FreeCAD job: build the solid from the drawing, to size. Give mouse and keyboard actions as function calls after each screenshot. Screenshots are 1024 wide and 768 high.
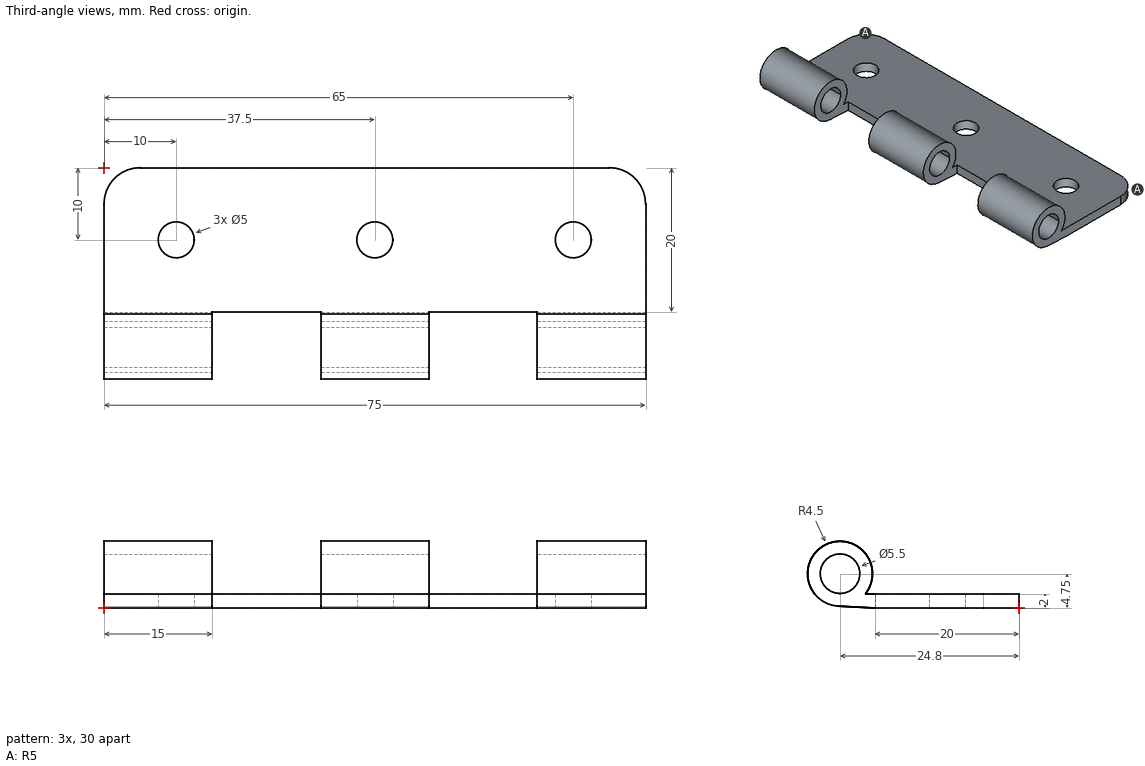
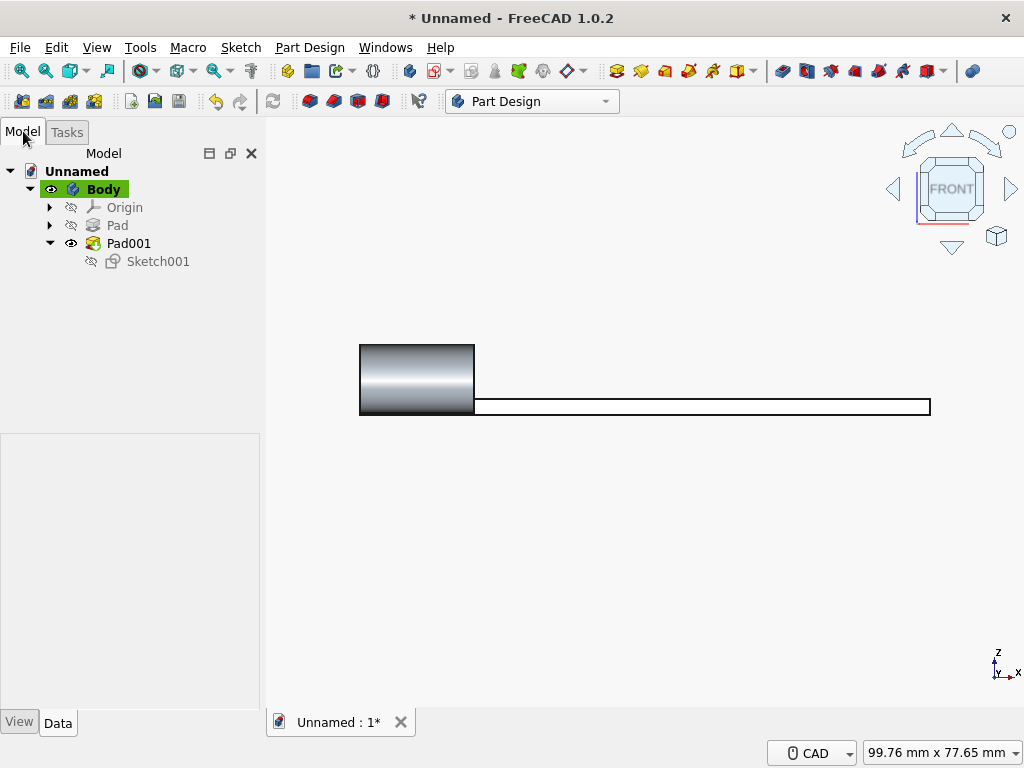
click(116, 243)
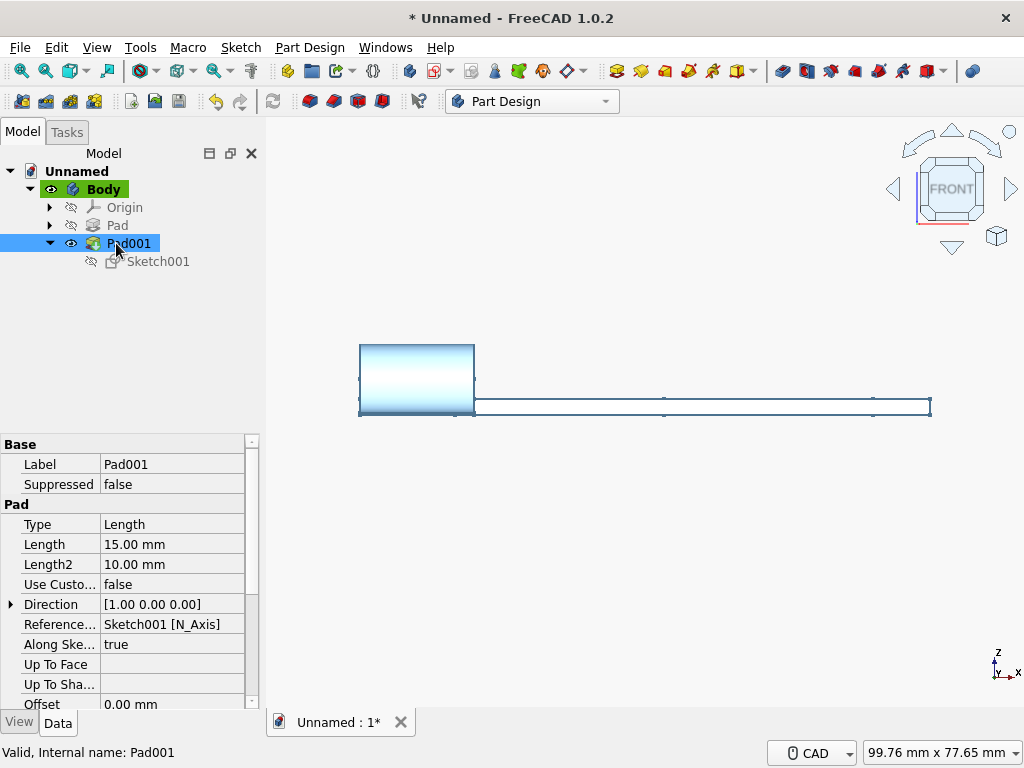
click(46, 102)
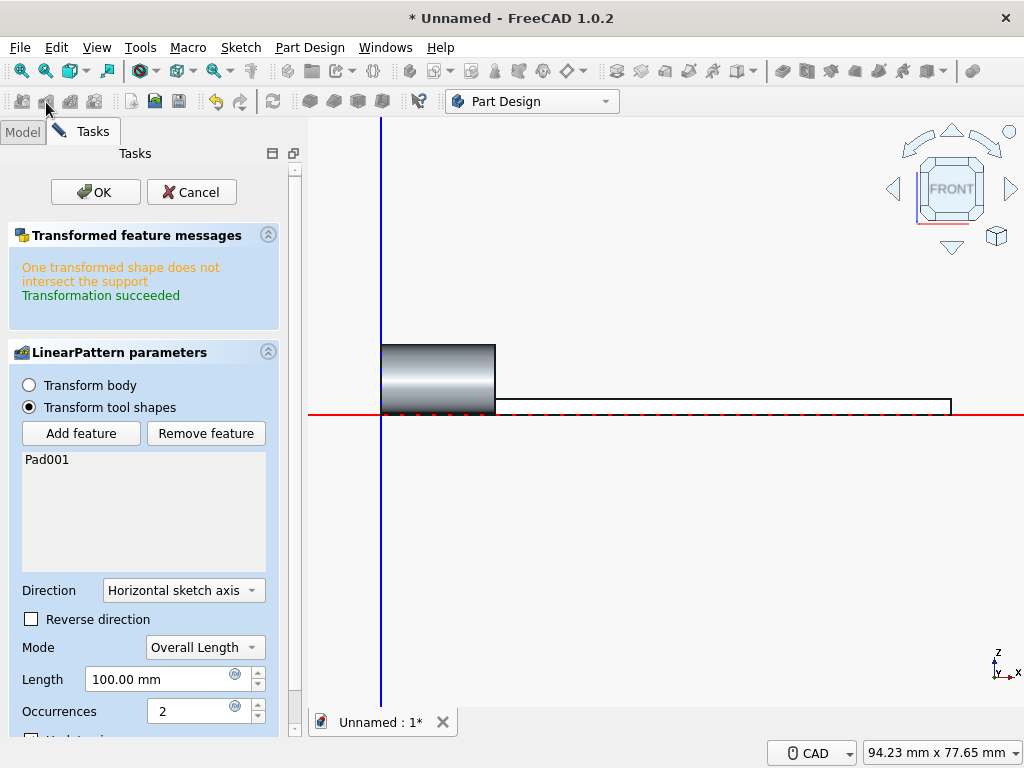
click(184, 590)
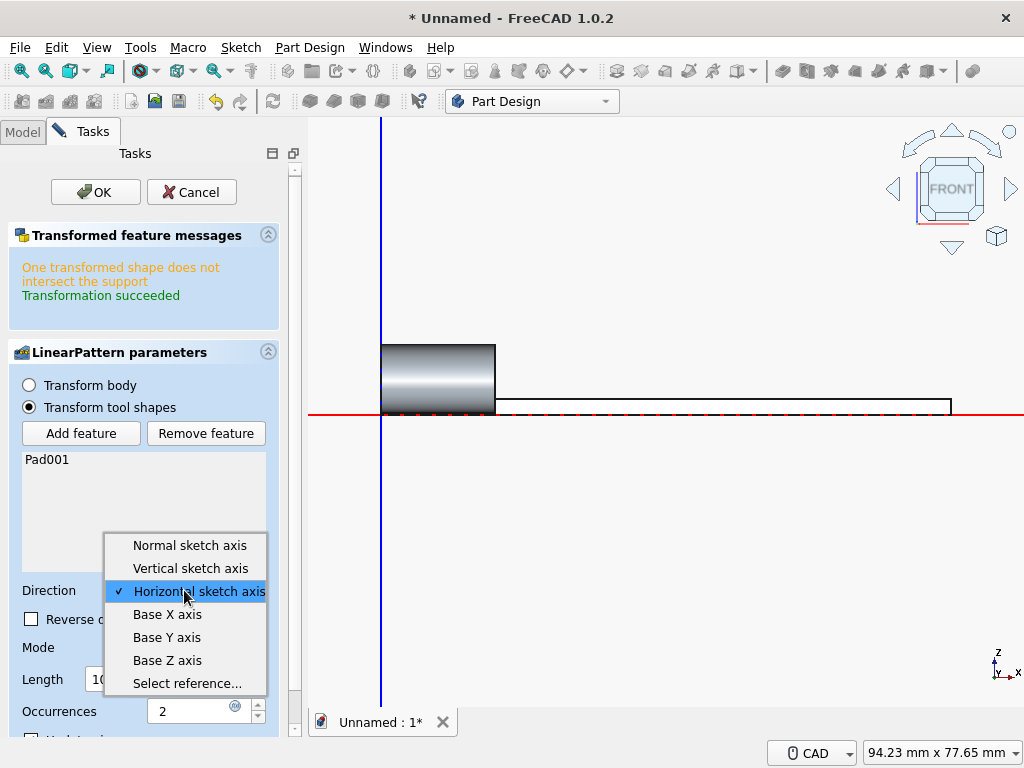
click(184, 614)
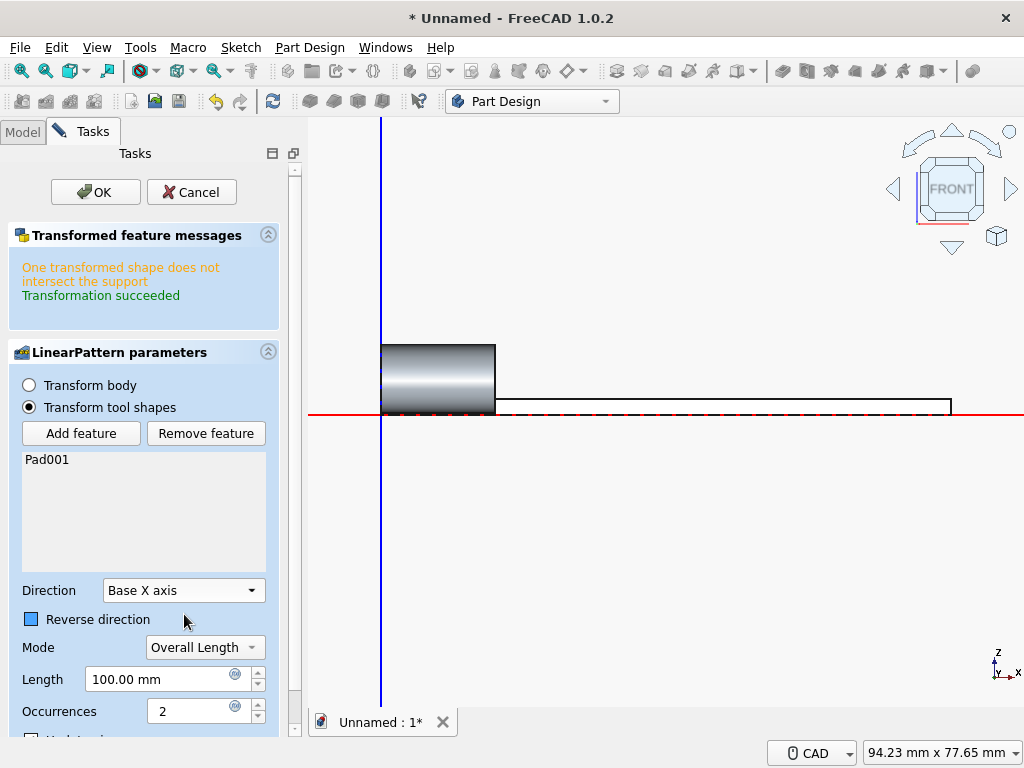
click(206, 648)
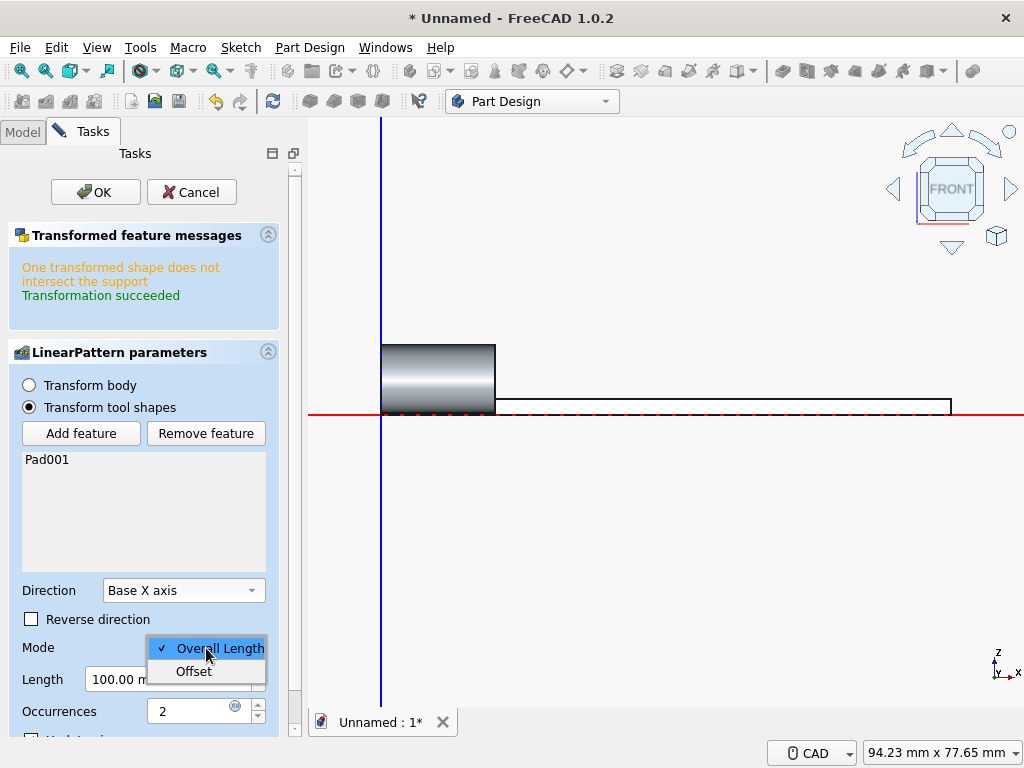
click(206, 672)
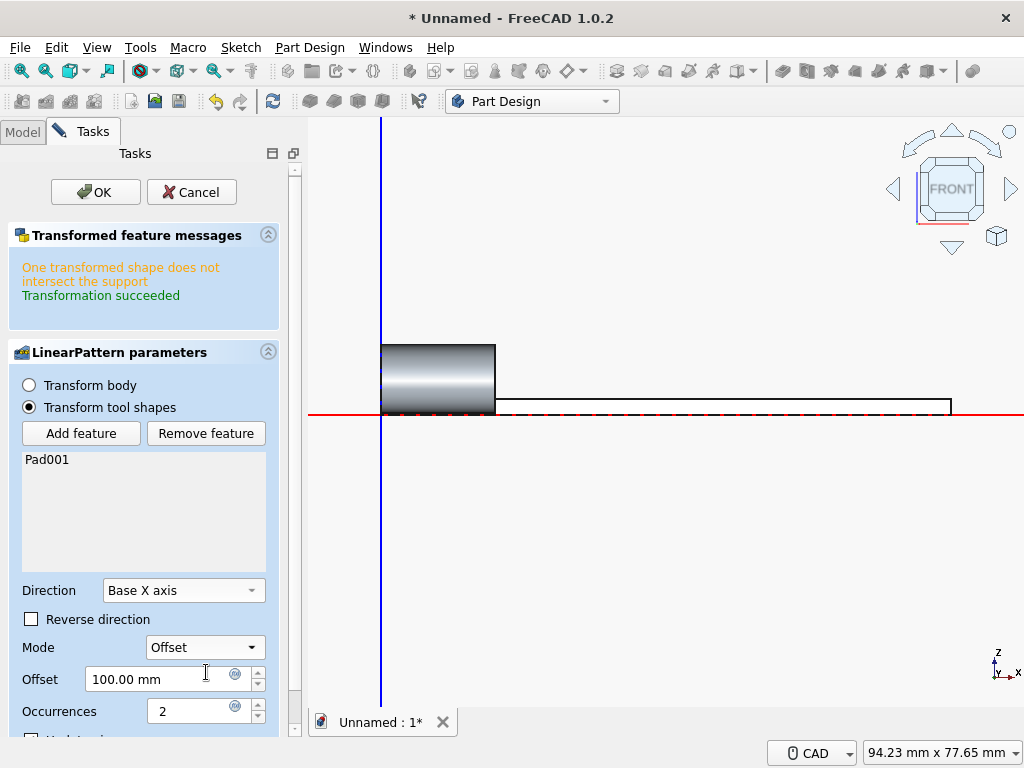
triple_click(168, 679)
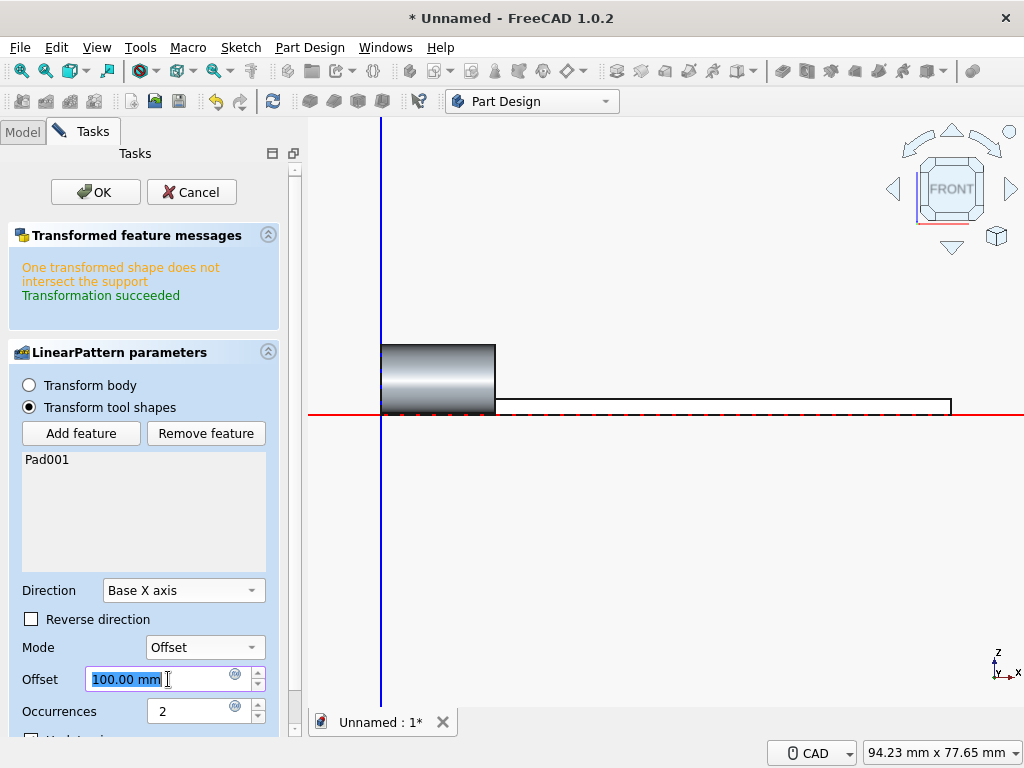
text(30)
key(Tab)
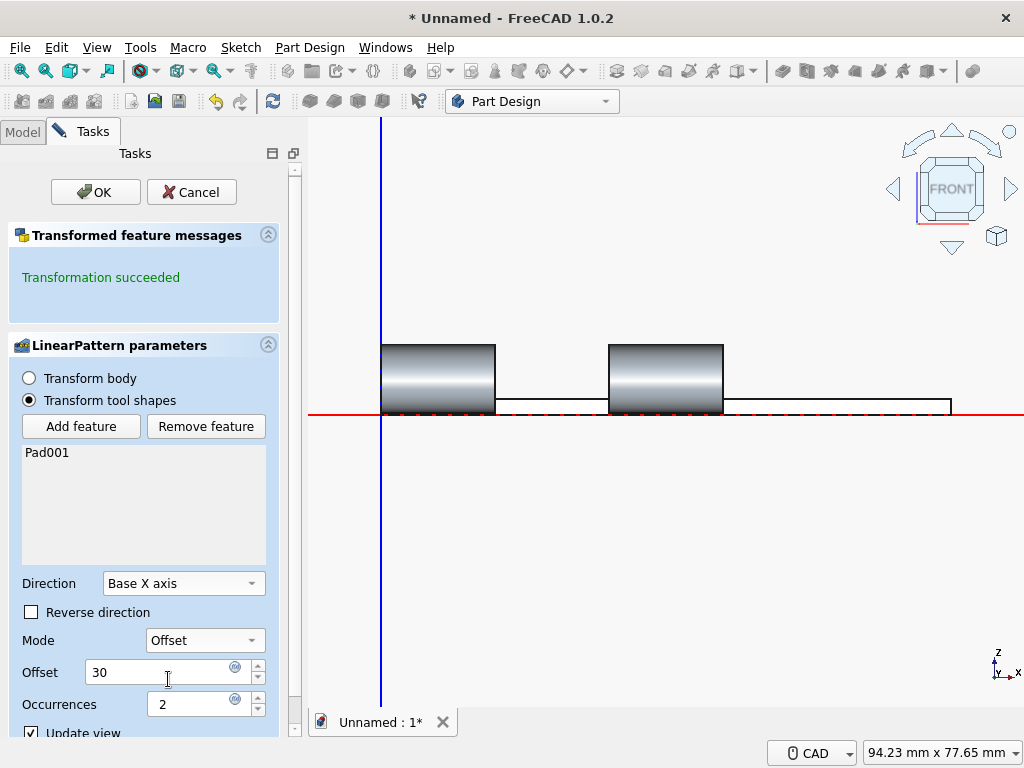
triple_click(198, 704)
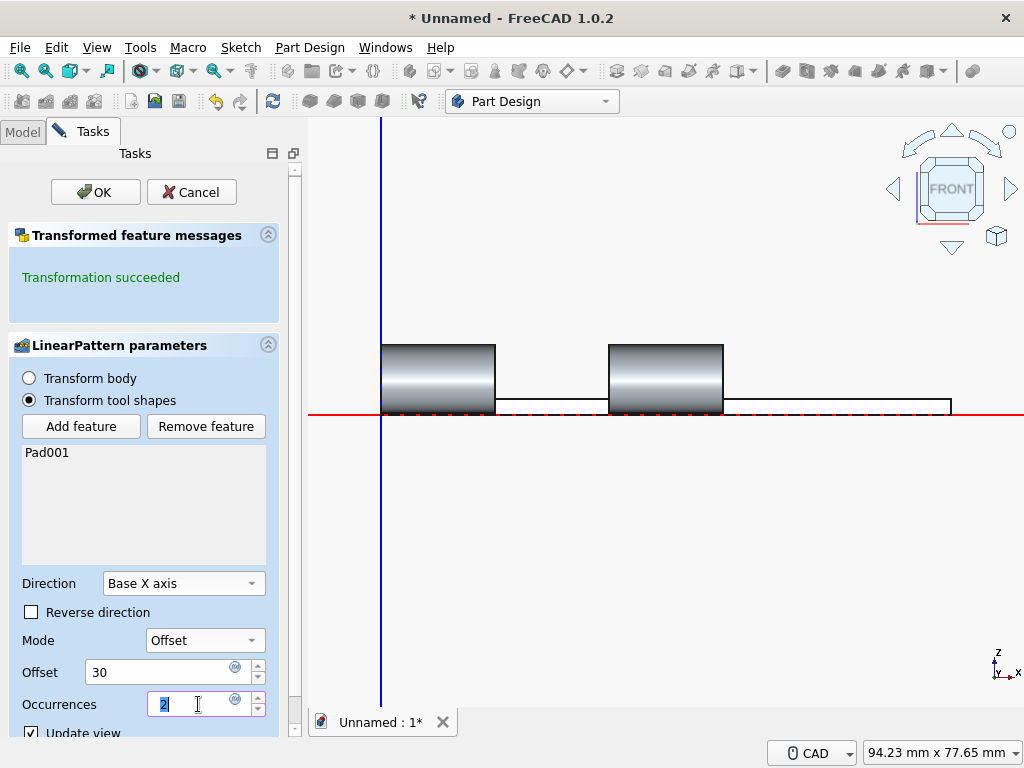
text(3)
key(Tab)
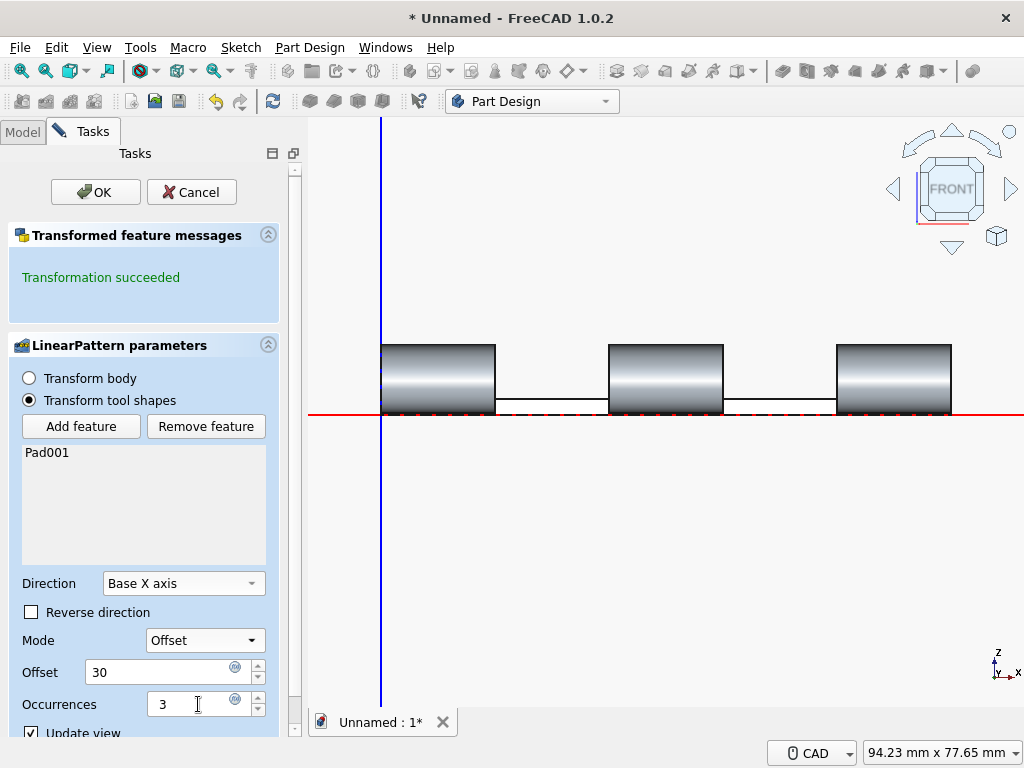
click(96, 192)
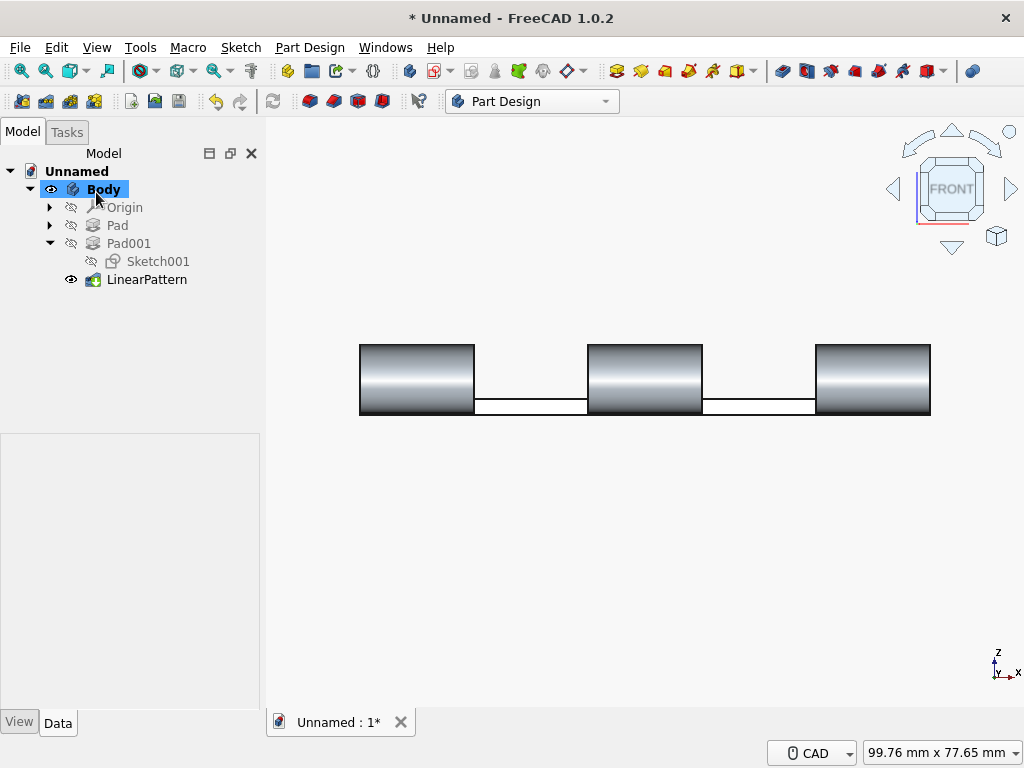
scroll(360, 406, up, 5)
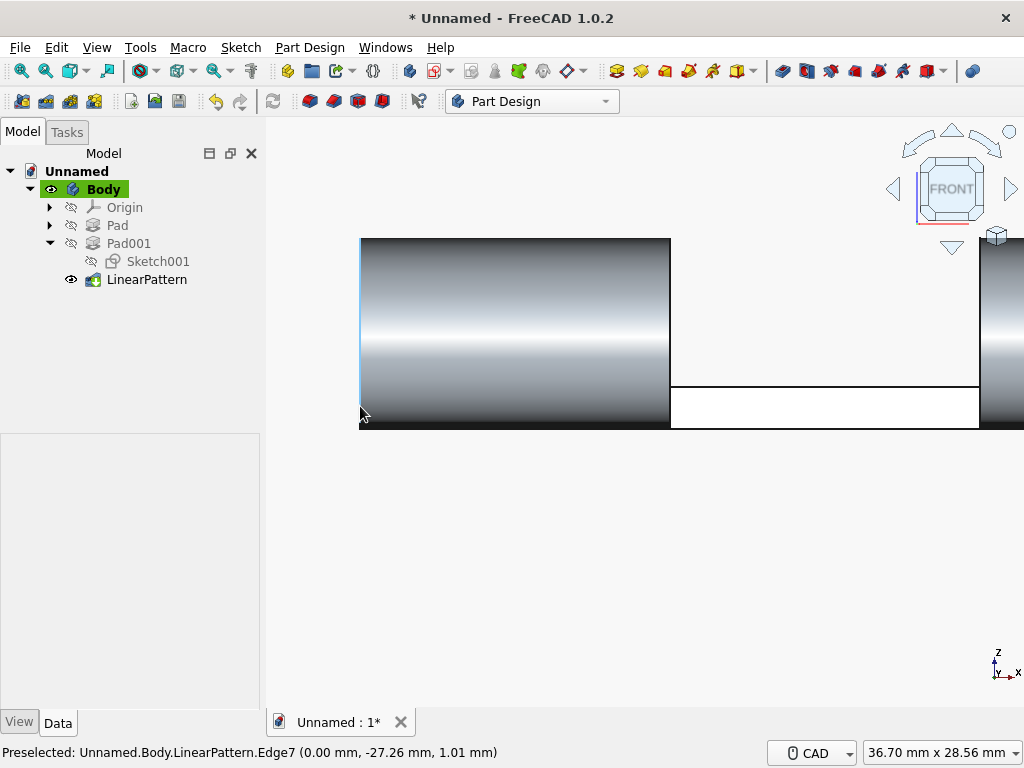
click(22, 72)